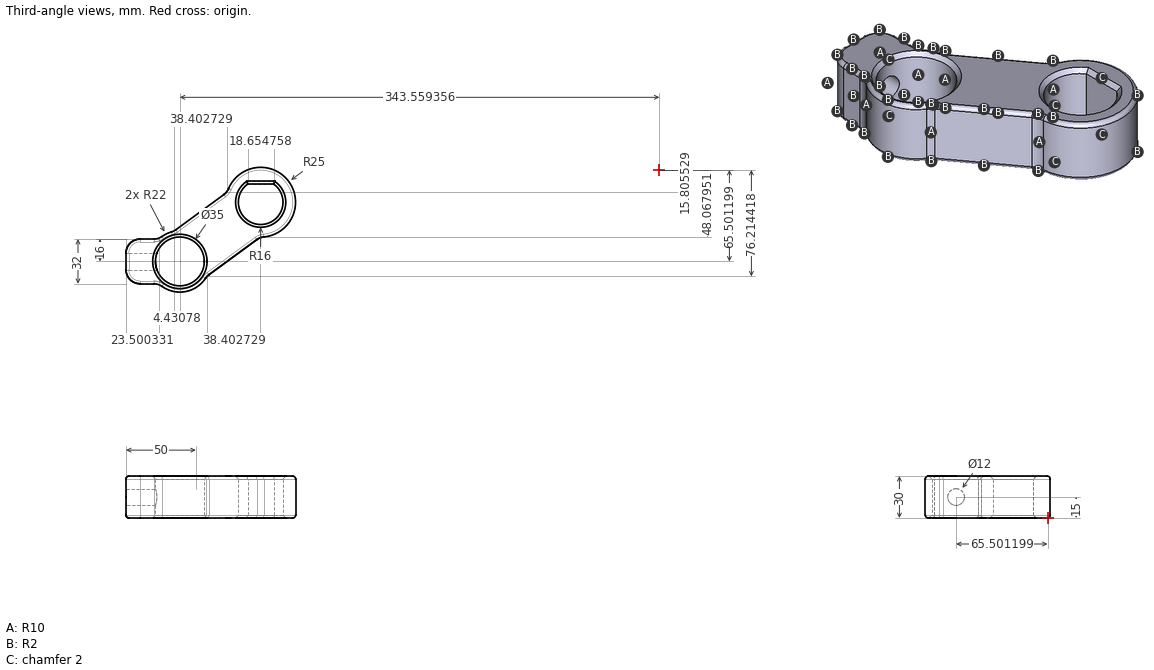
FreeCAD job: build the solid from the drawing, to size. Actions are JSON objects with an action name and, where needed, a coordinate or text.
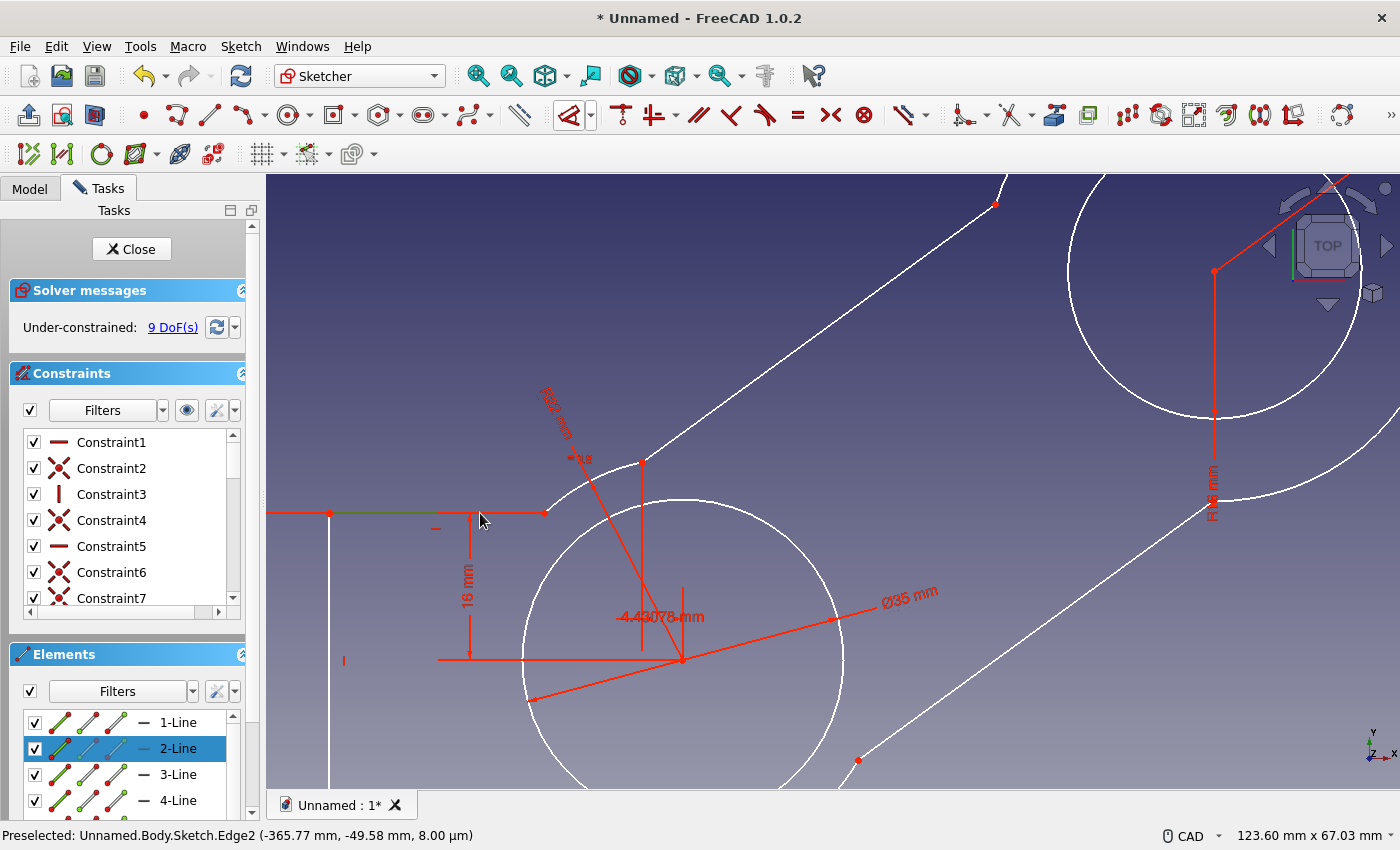
{"action": "key", "text": "l"}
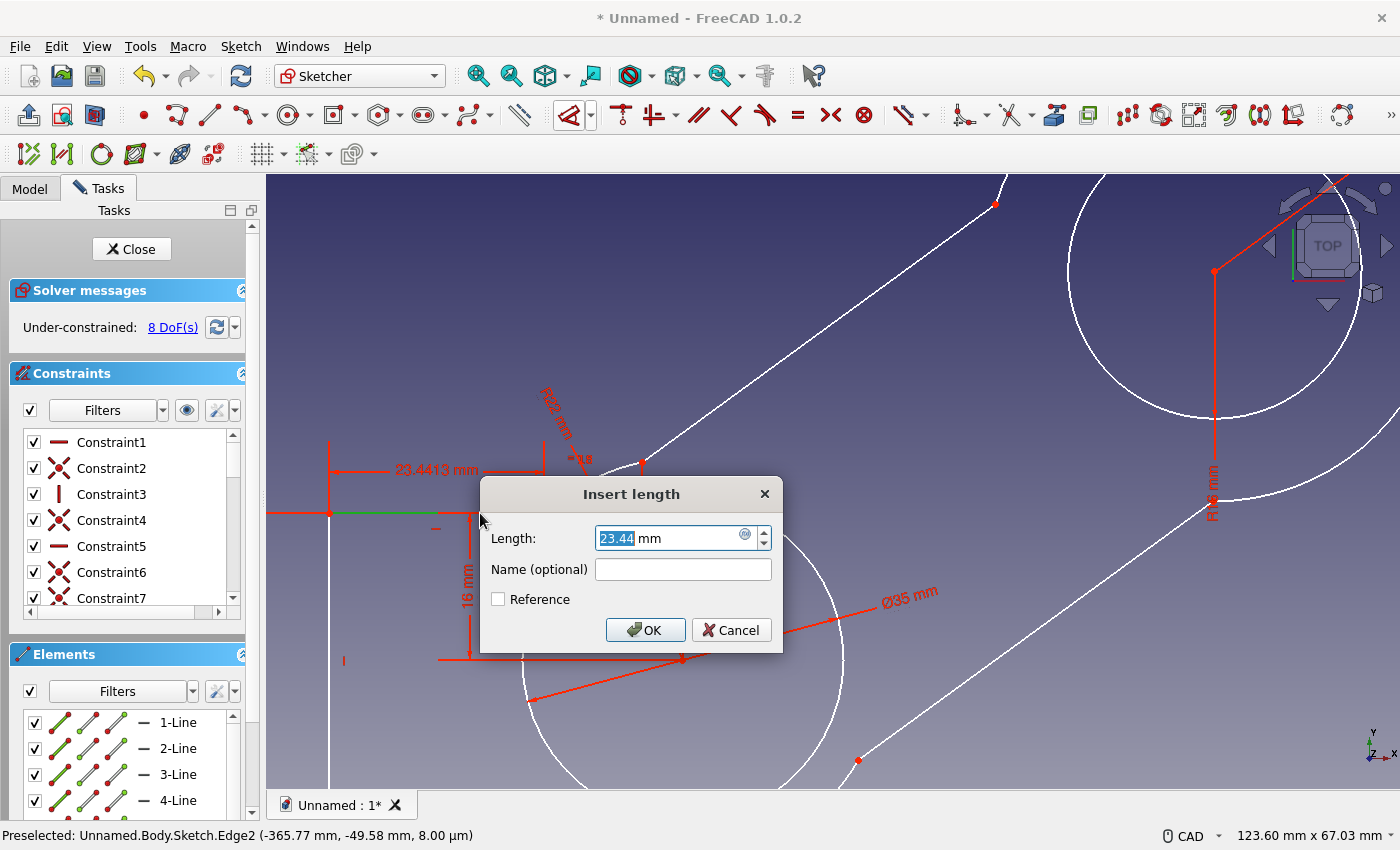
{"action": "type", "text": "23.500331"}
{"action": "key", "text": "Return"}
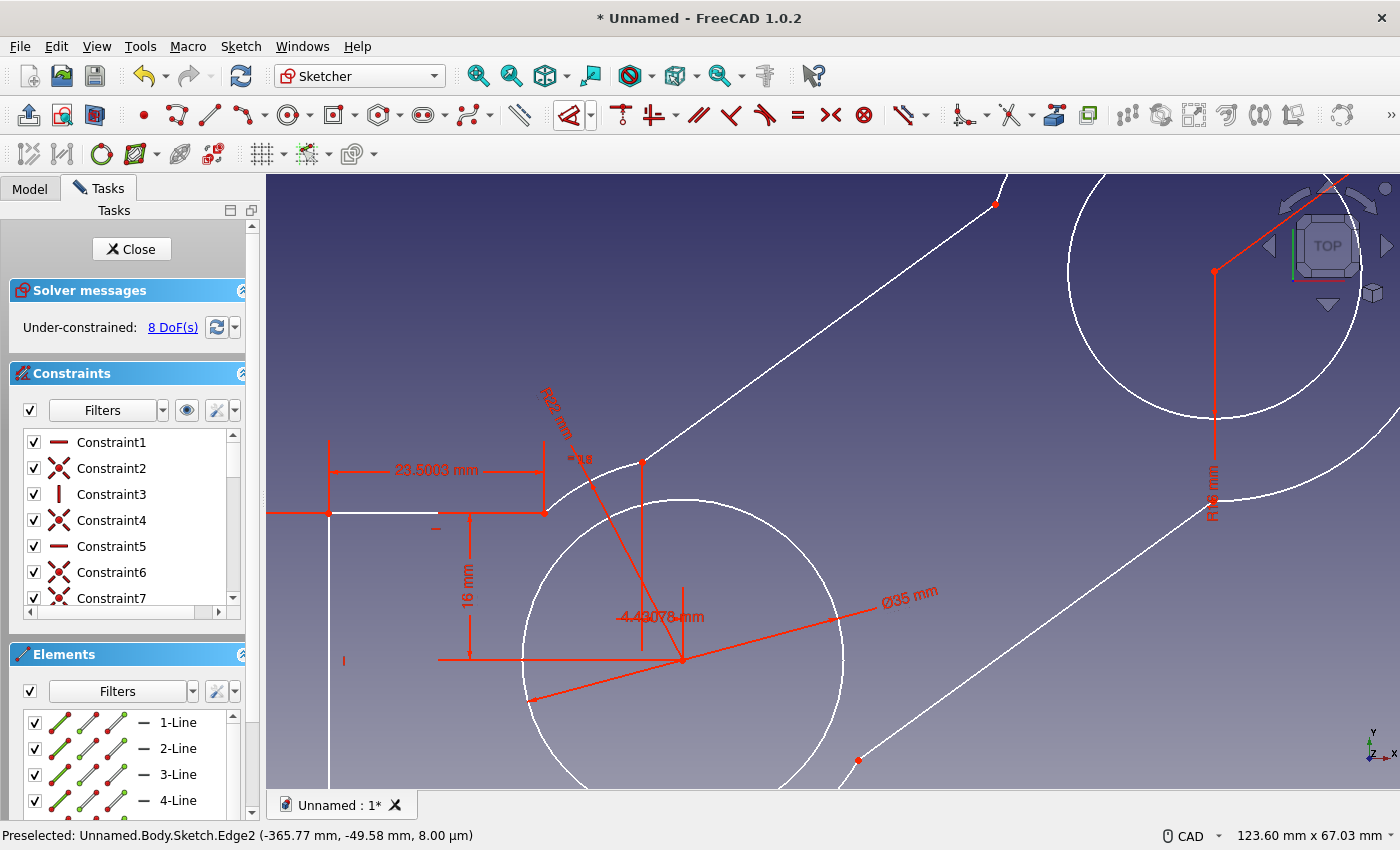
{"action": "scroll", "coordinate": [643, 463], "scroll_direction": "down", "scroll_amount": 3}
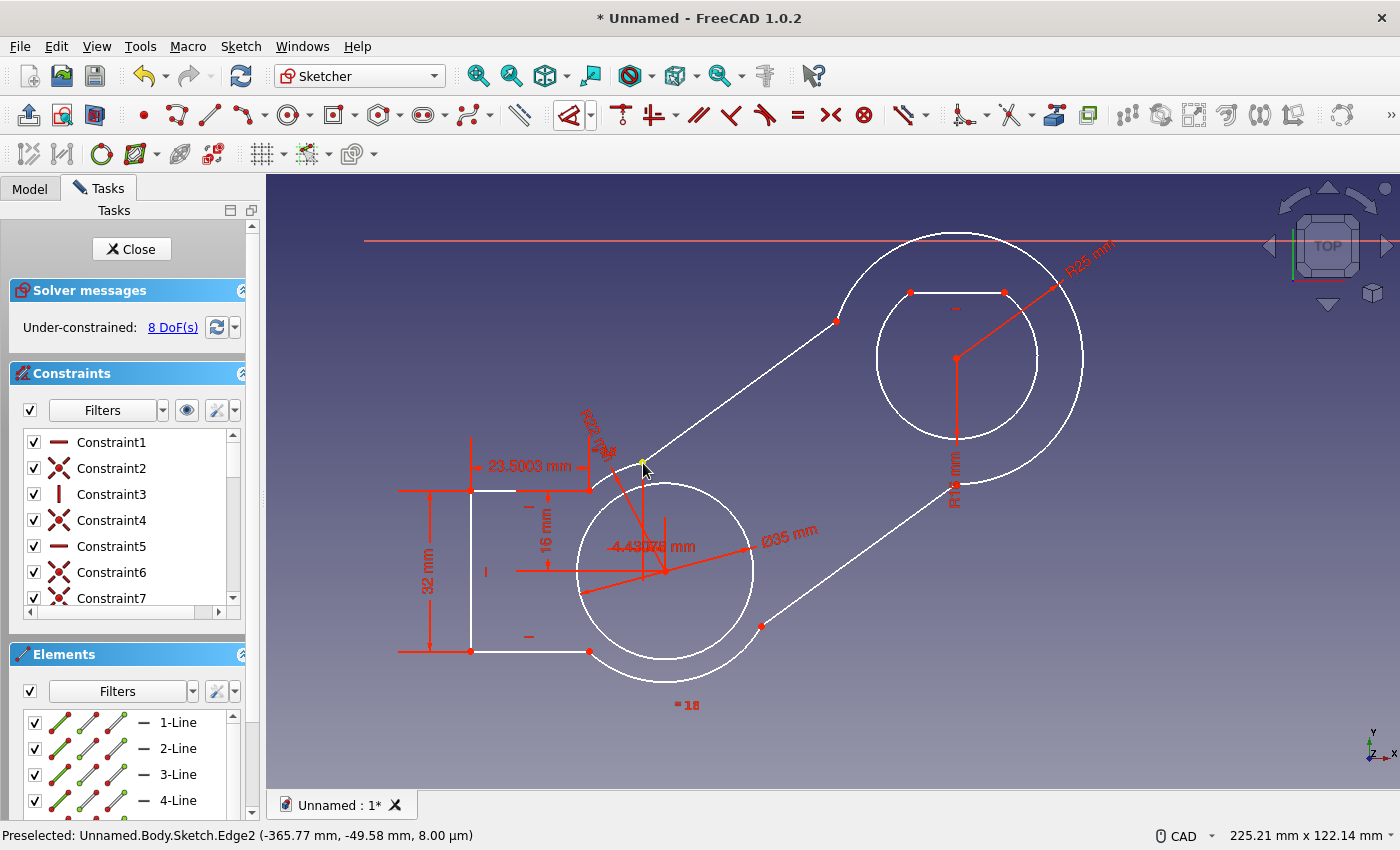
{"action": "left_click", "coordinate": [976, 293]}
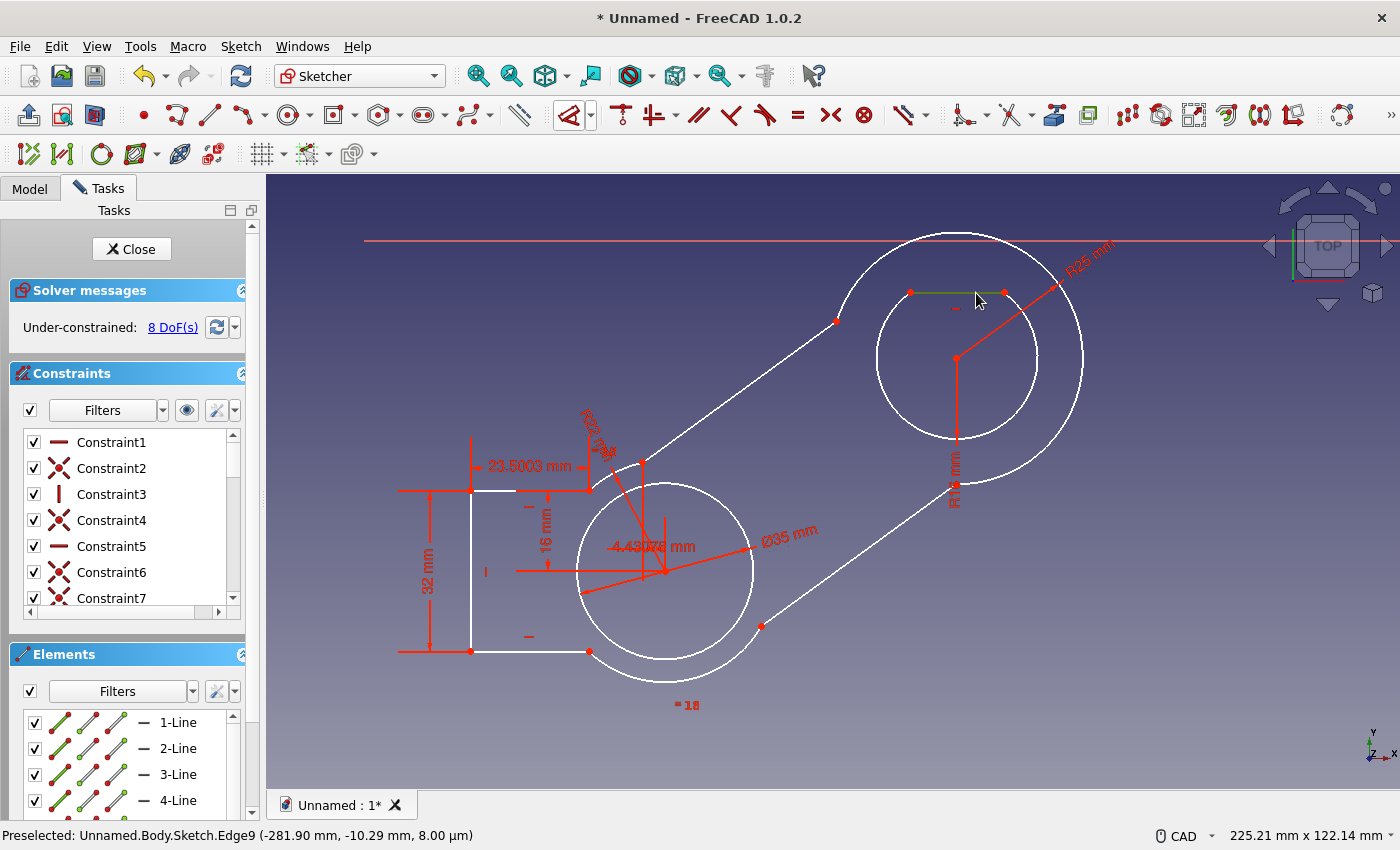
{"action": "key", "text": "l"}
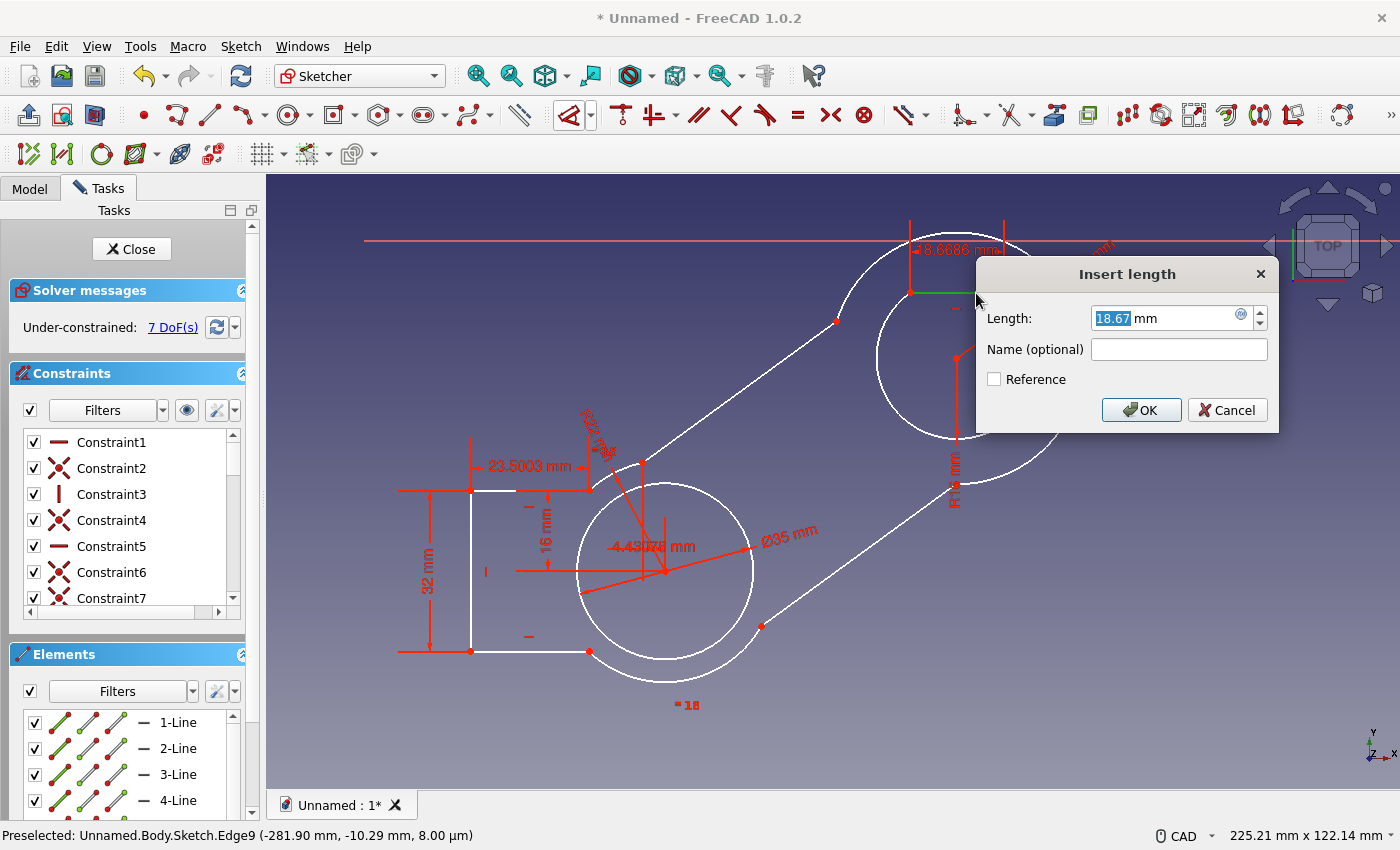
{"action": "type", "text": "18.654758"}
{"action": "key", "text": "Return"}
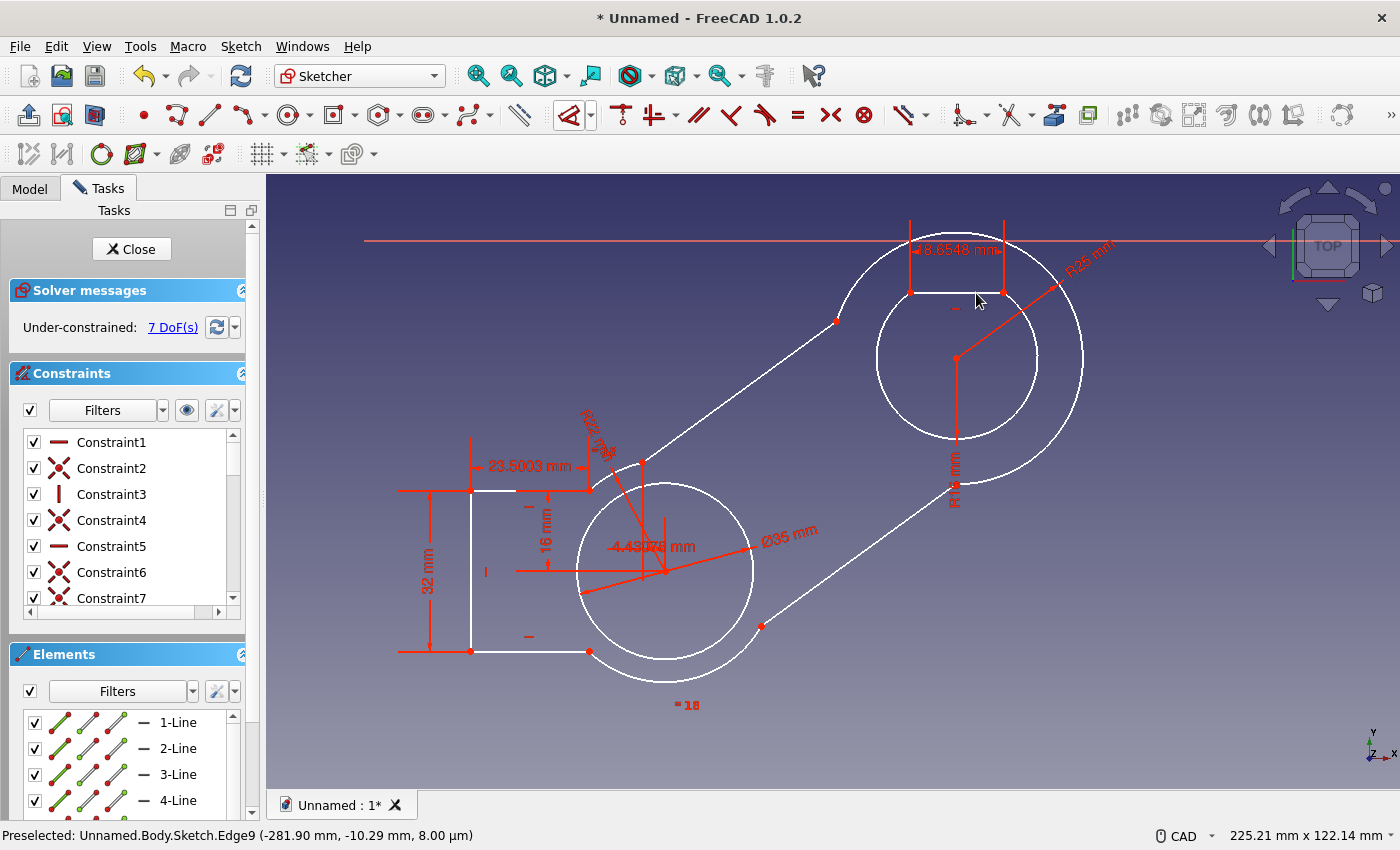
{"action": "left_click", "coordinate": [665, 571]}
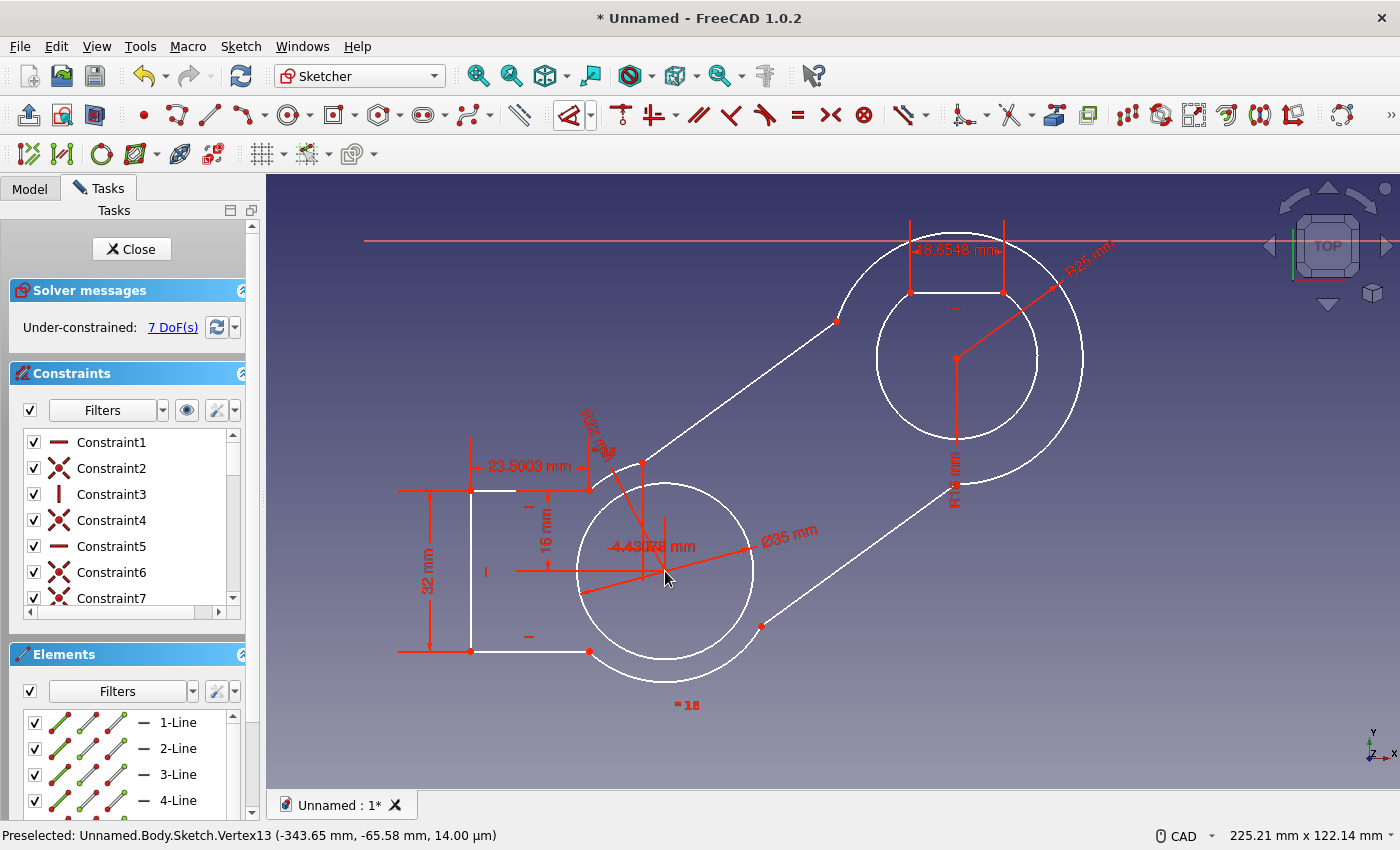
{"action": "key", "text": "i"}